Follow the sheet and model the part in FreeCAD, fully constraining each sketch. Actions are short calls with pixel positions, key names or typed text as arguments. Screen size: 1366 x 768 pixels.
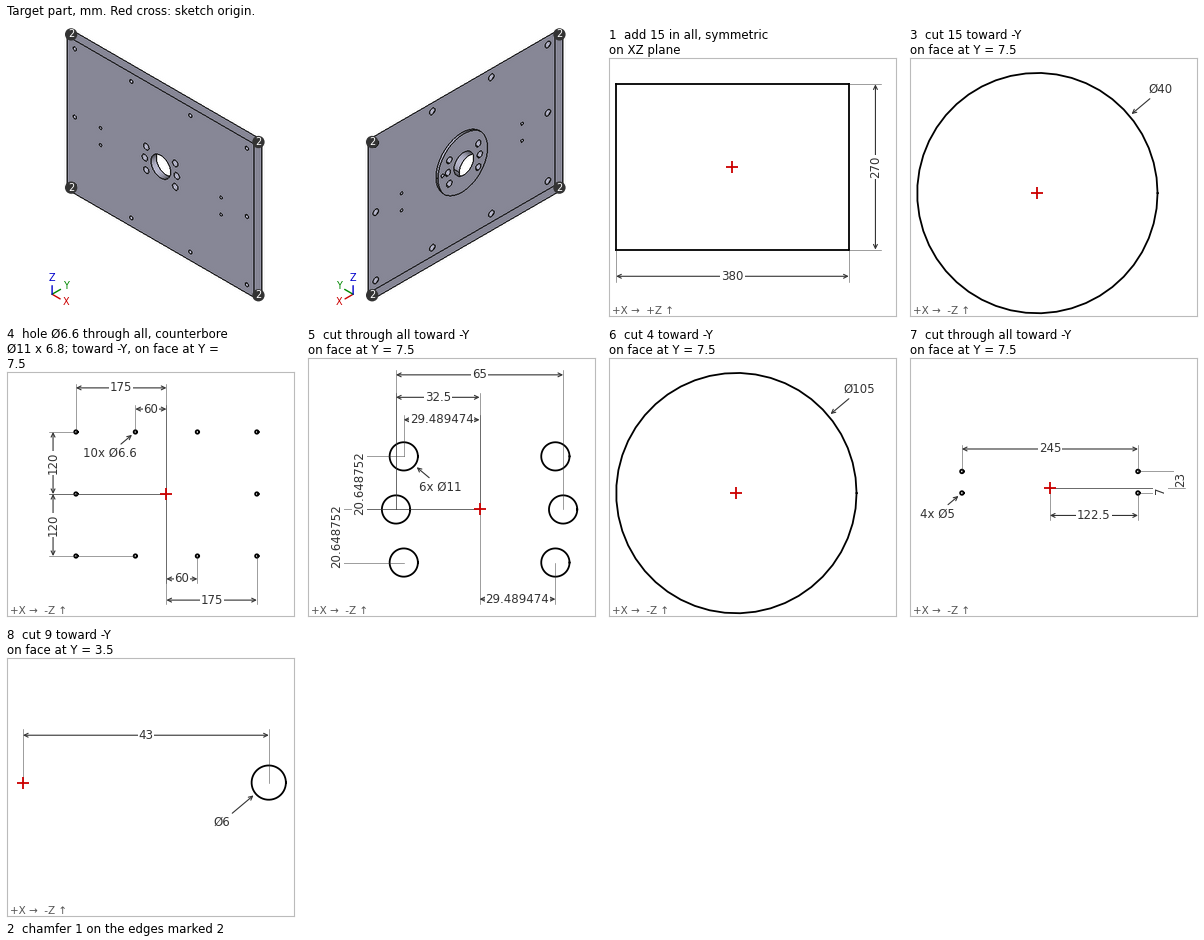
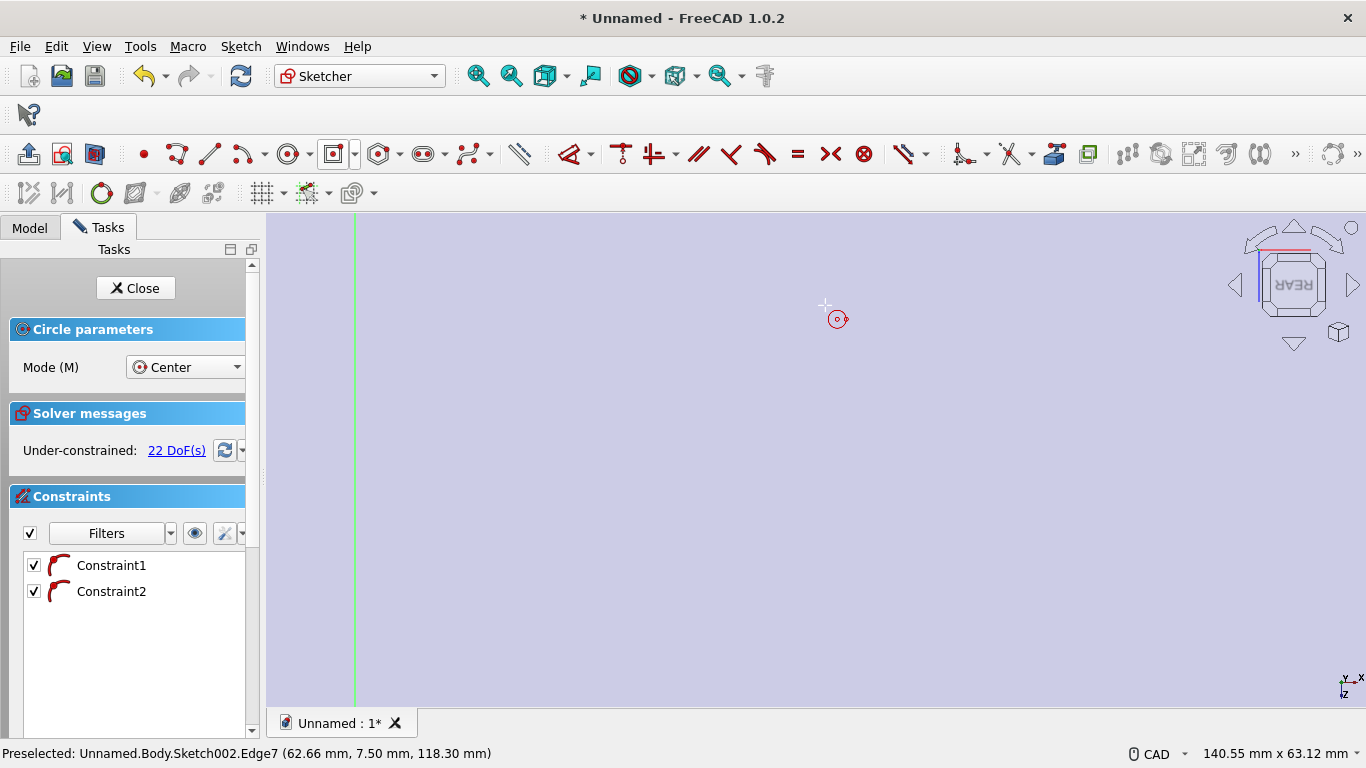
scroll(825, 305, down, 9)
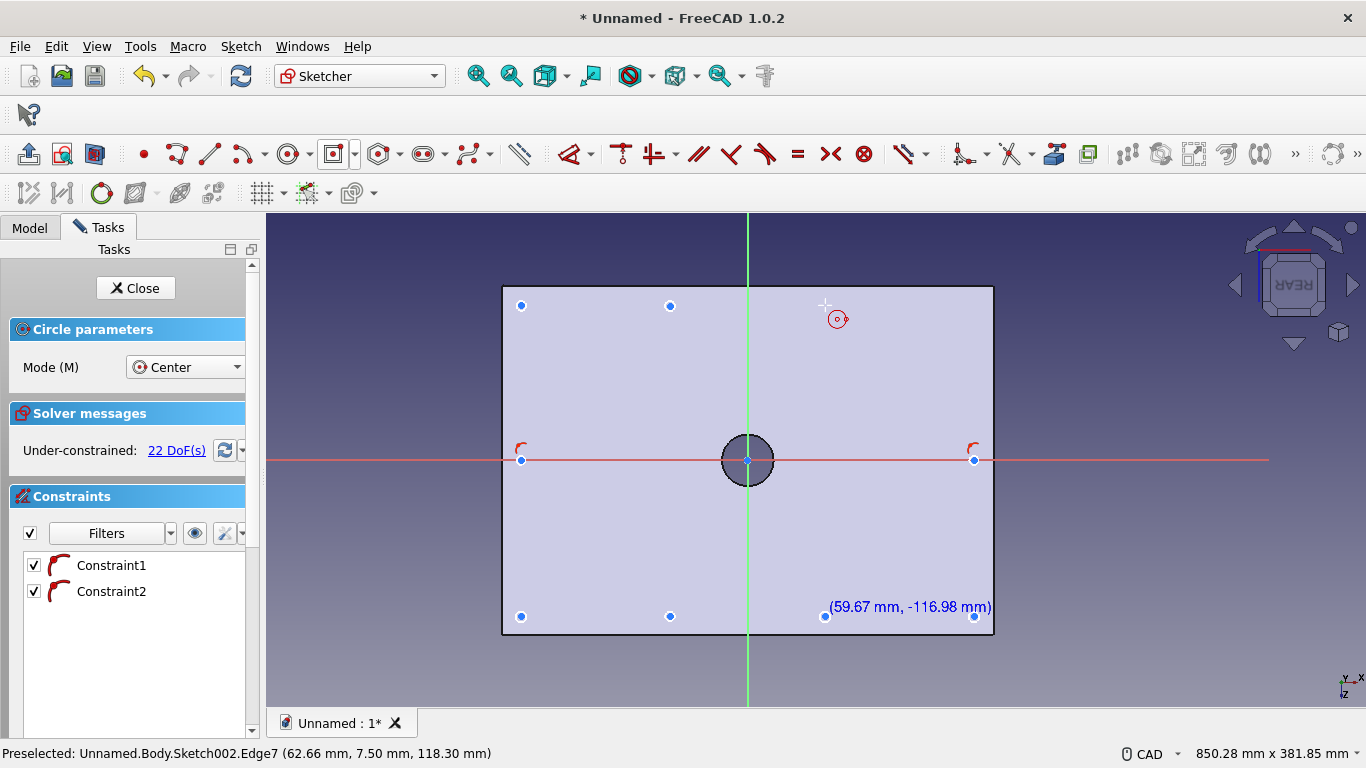
click(825, 305)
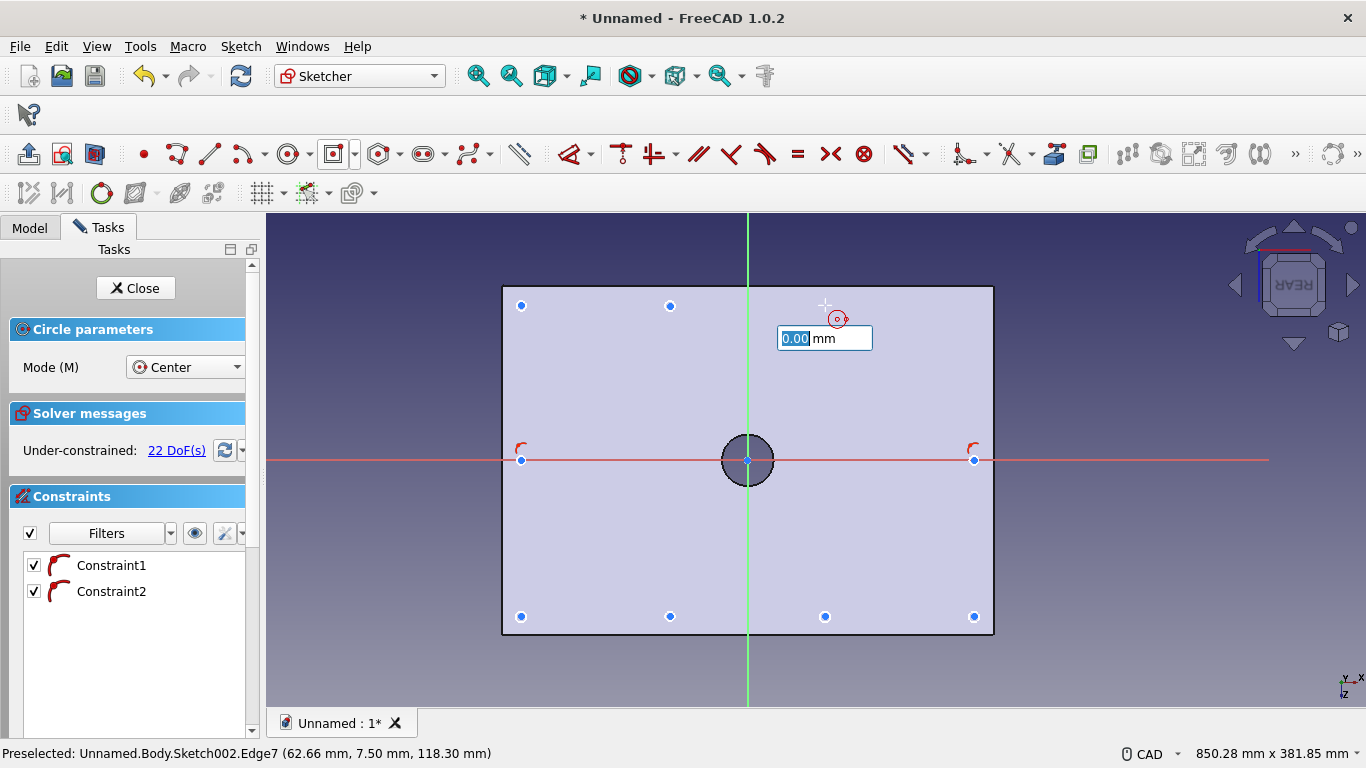
scroll(828, 302, up, 7)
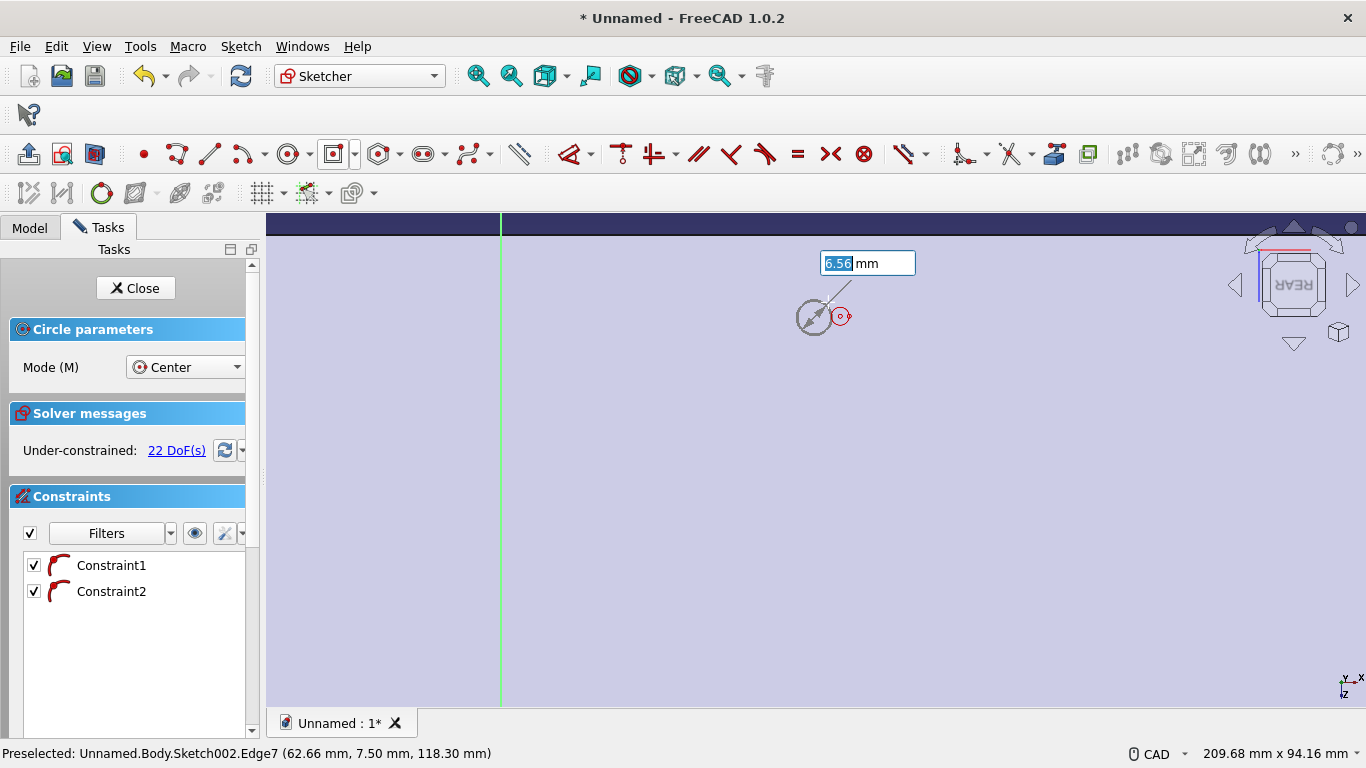
click(828, 302)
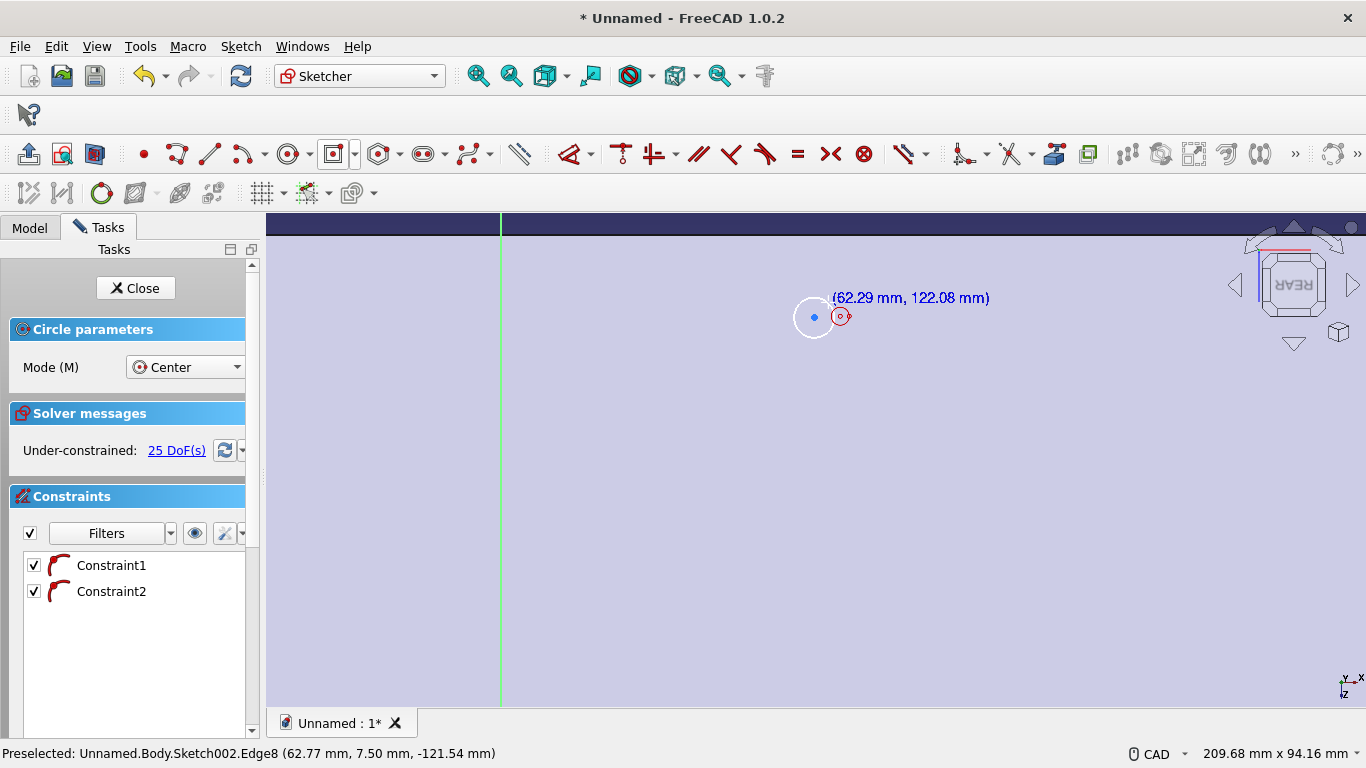
scroll(828, 302, down, 7)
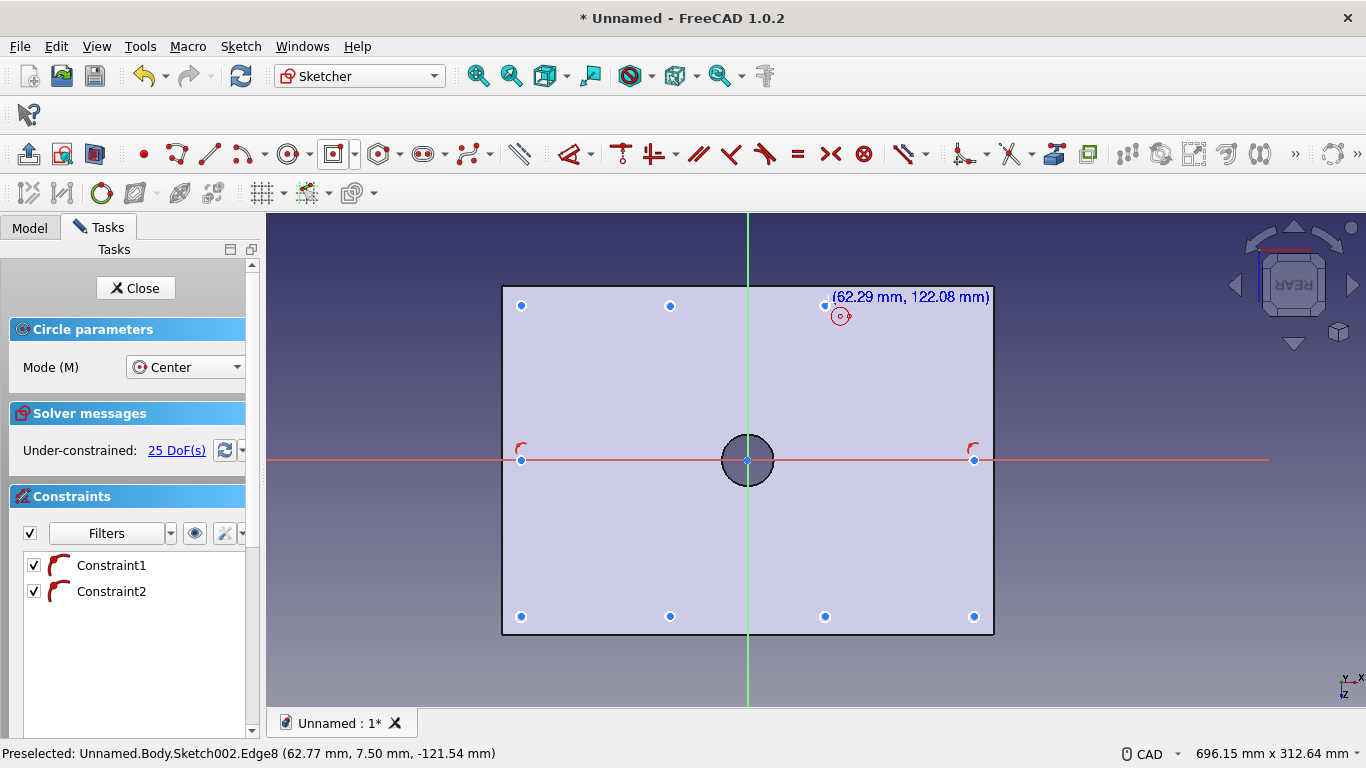
scroll(974, 305, up, 9)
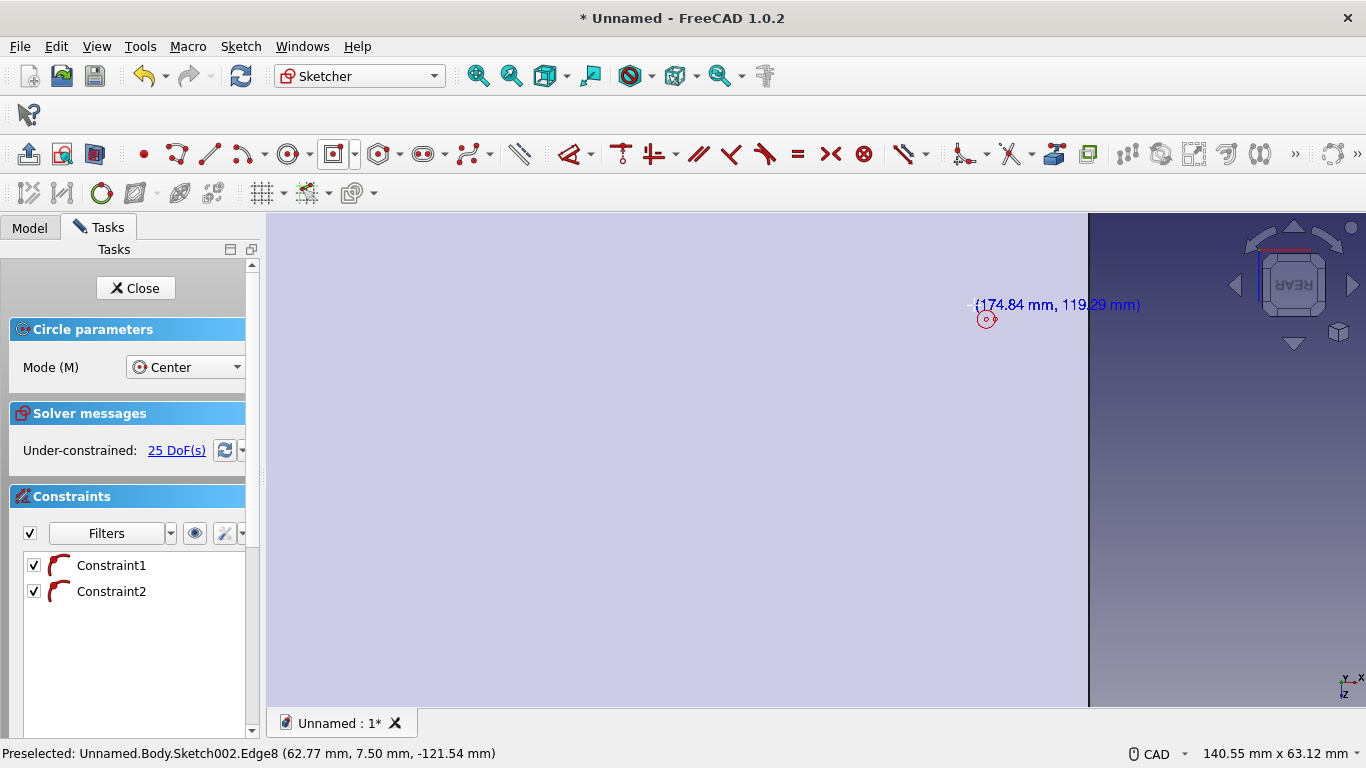
scroll(974, 305, down, 9)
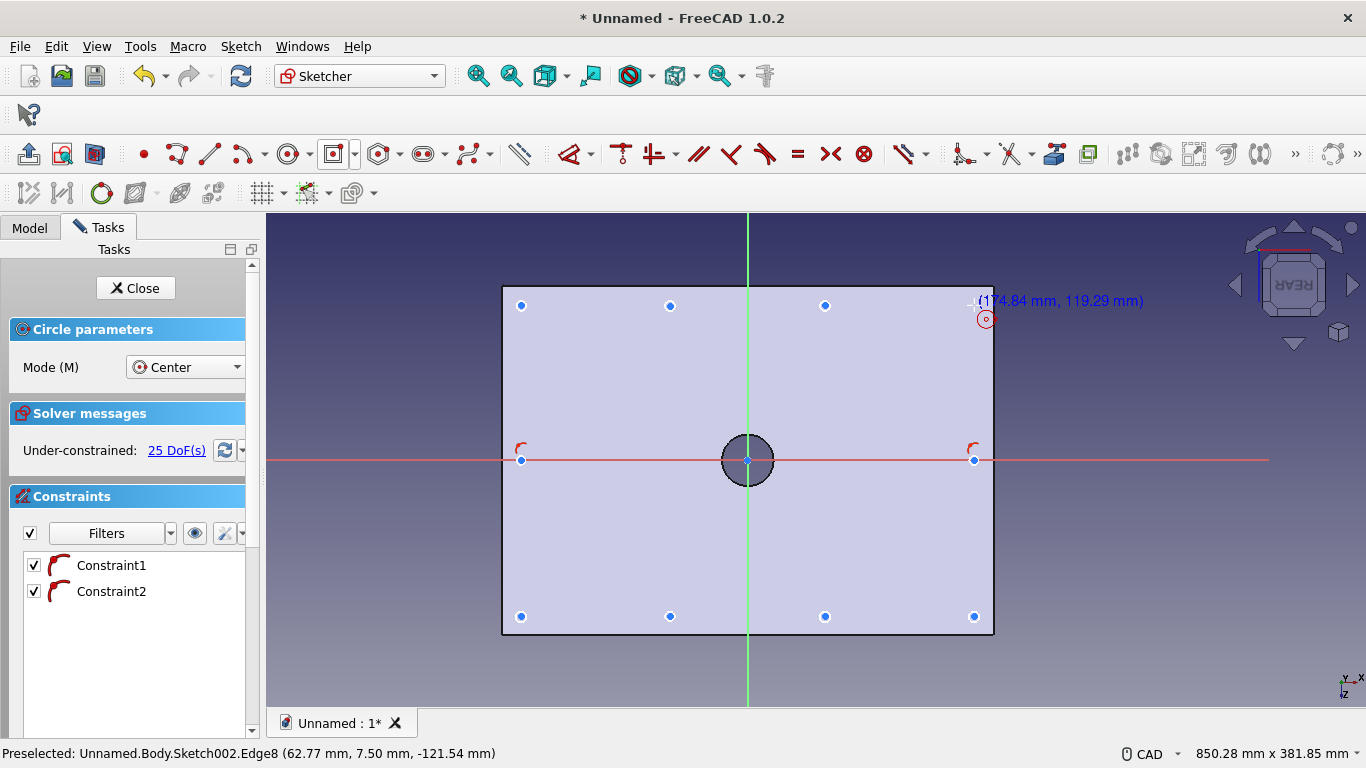
click(974, 305)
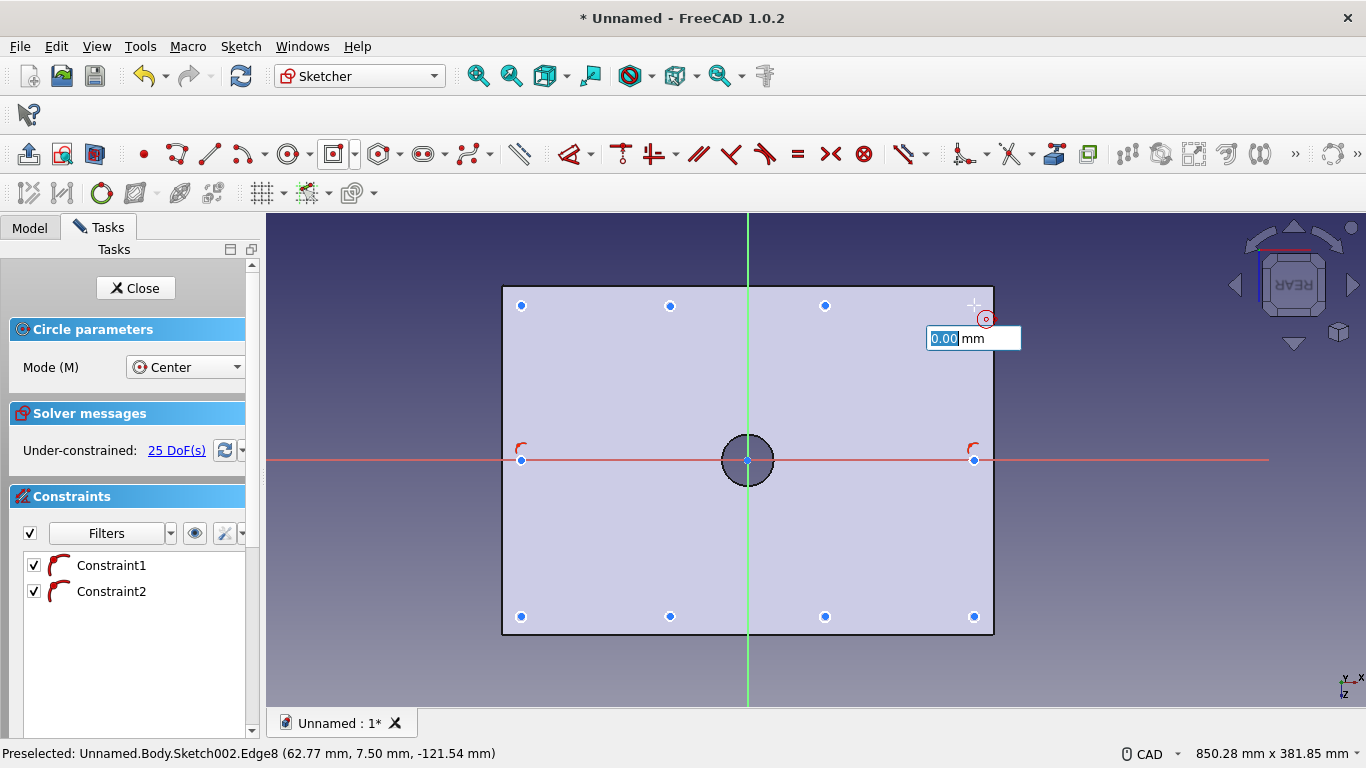
scroll(977, 302, up, 7)